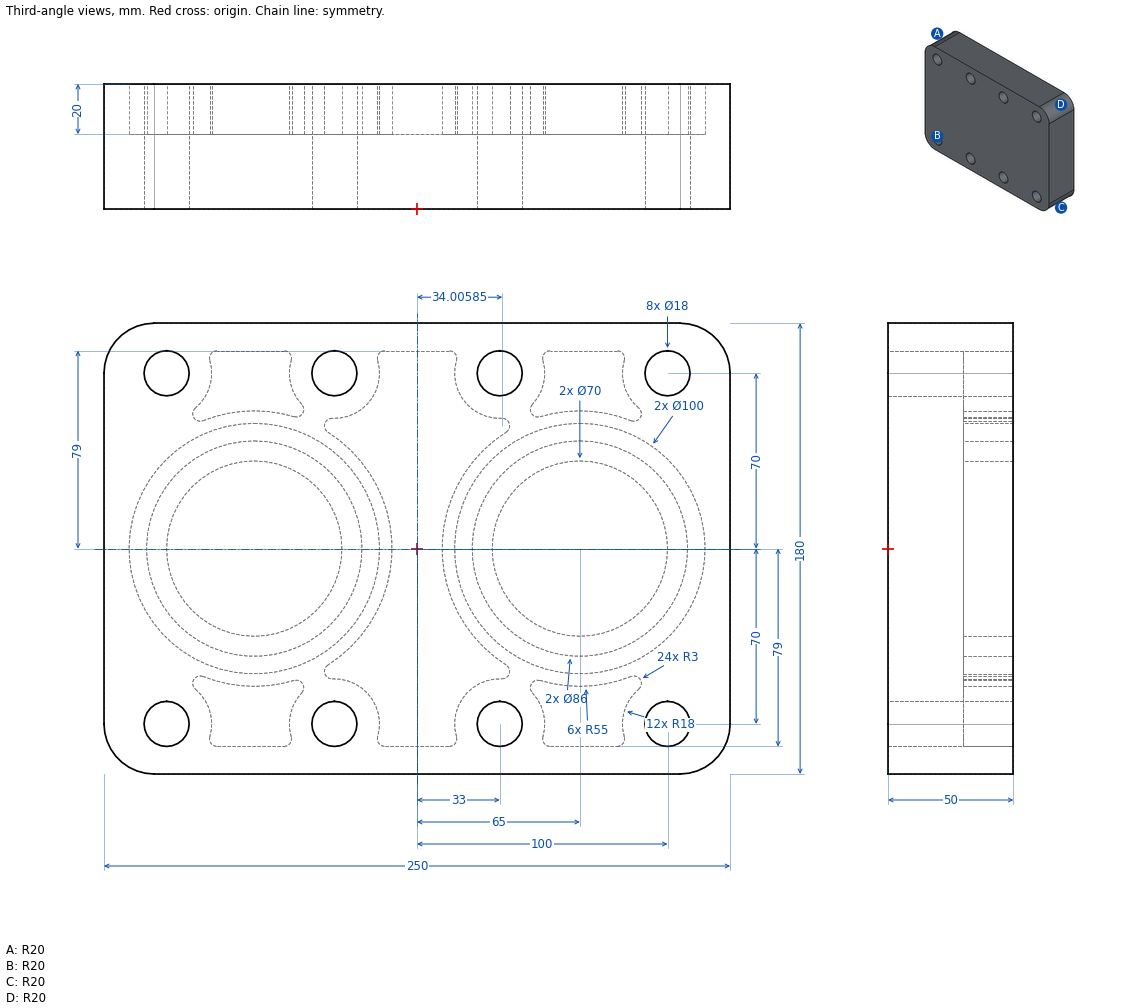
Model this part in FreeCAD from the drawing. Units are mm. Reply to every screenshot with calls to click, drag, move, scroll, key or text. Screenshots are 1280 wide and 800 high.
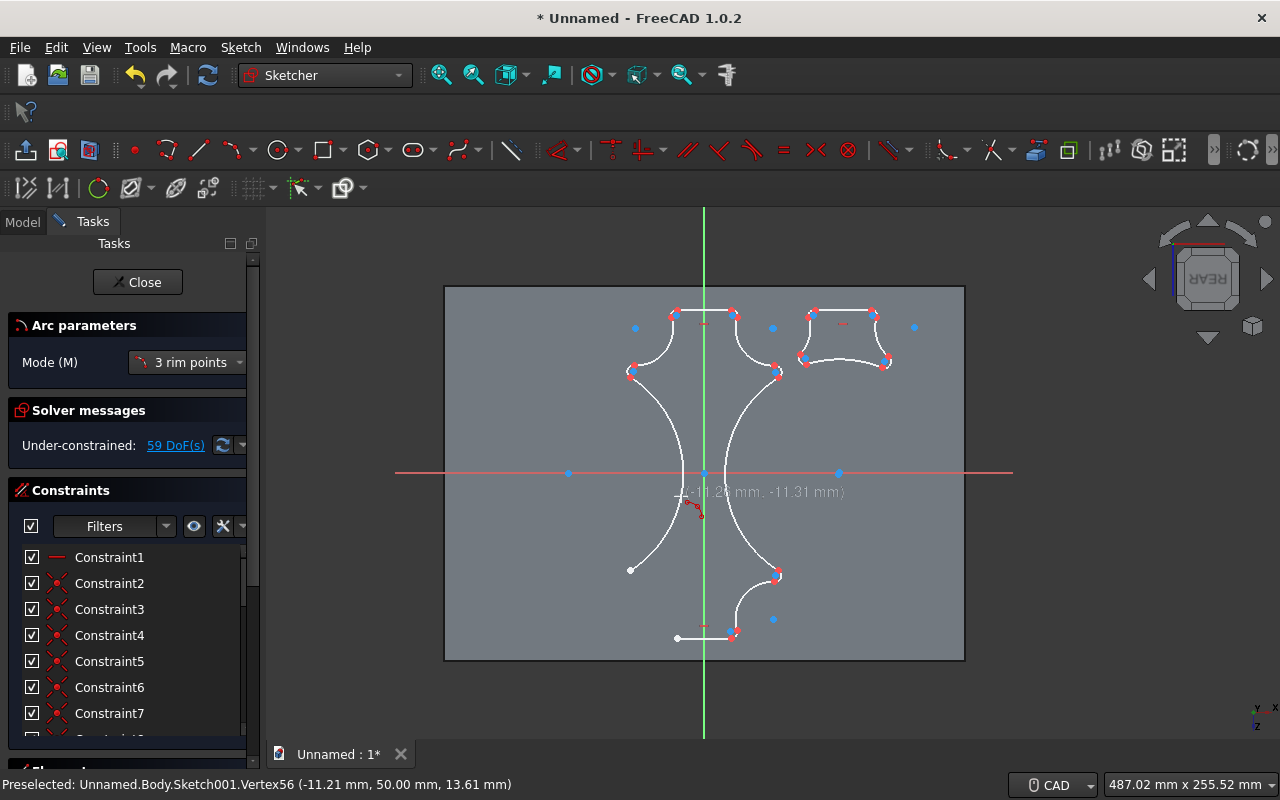
click(630, 571)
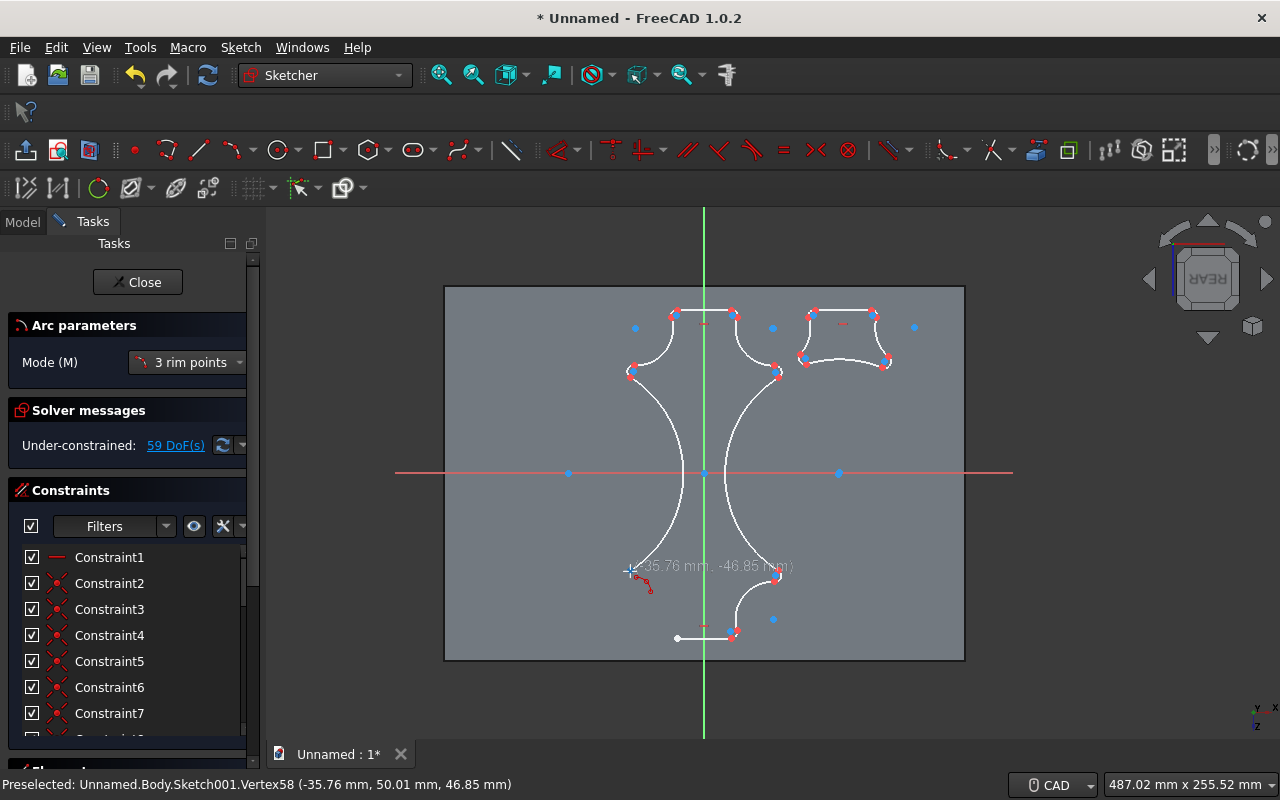
scroll(634, 582, up, 2)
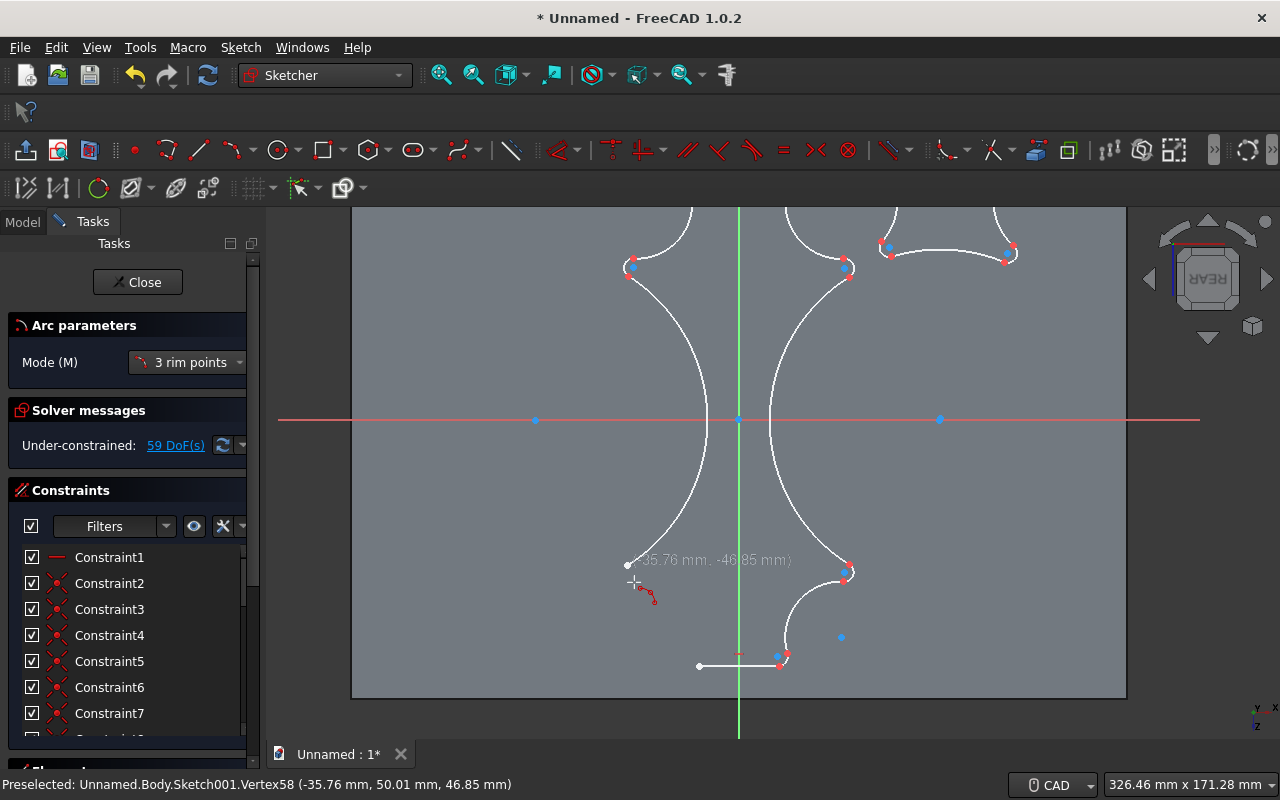
click(634, 581)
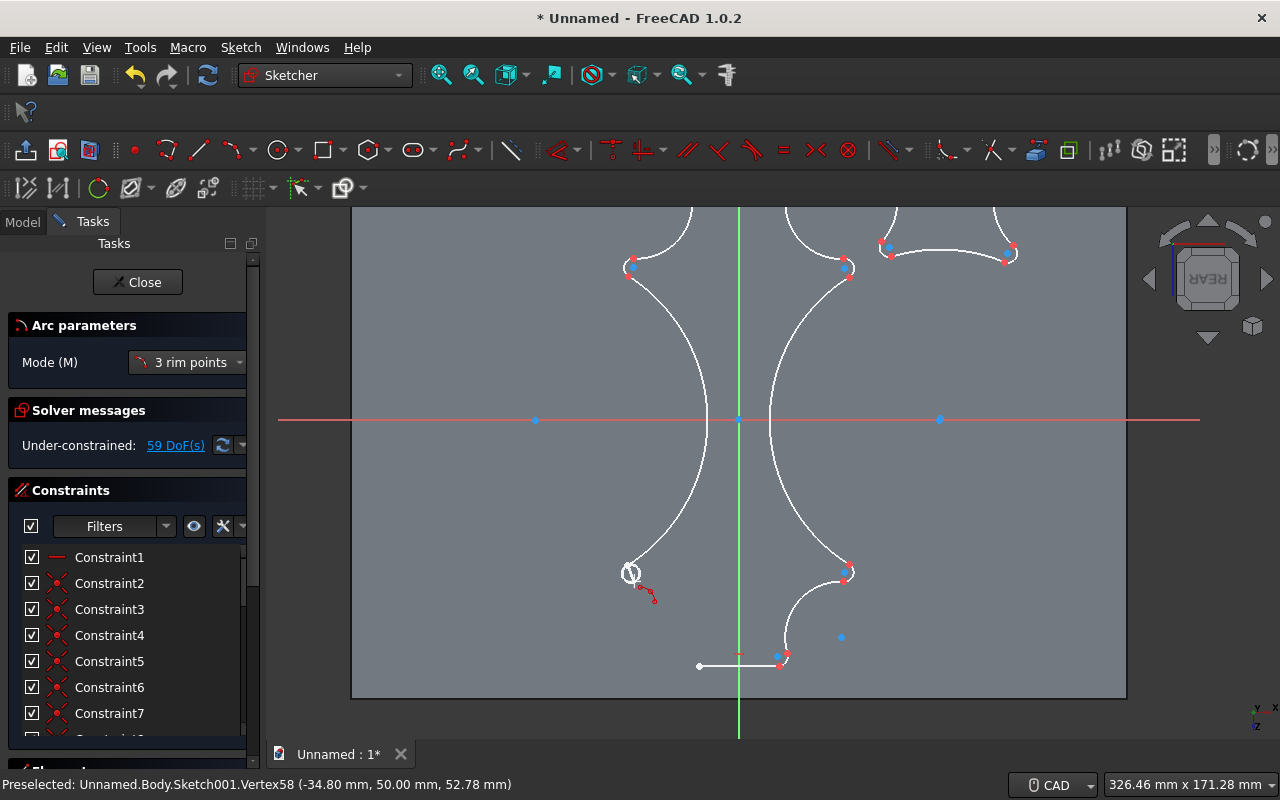
scroll(624, 575, up, 5)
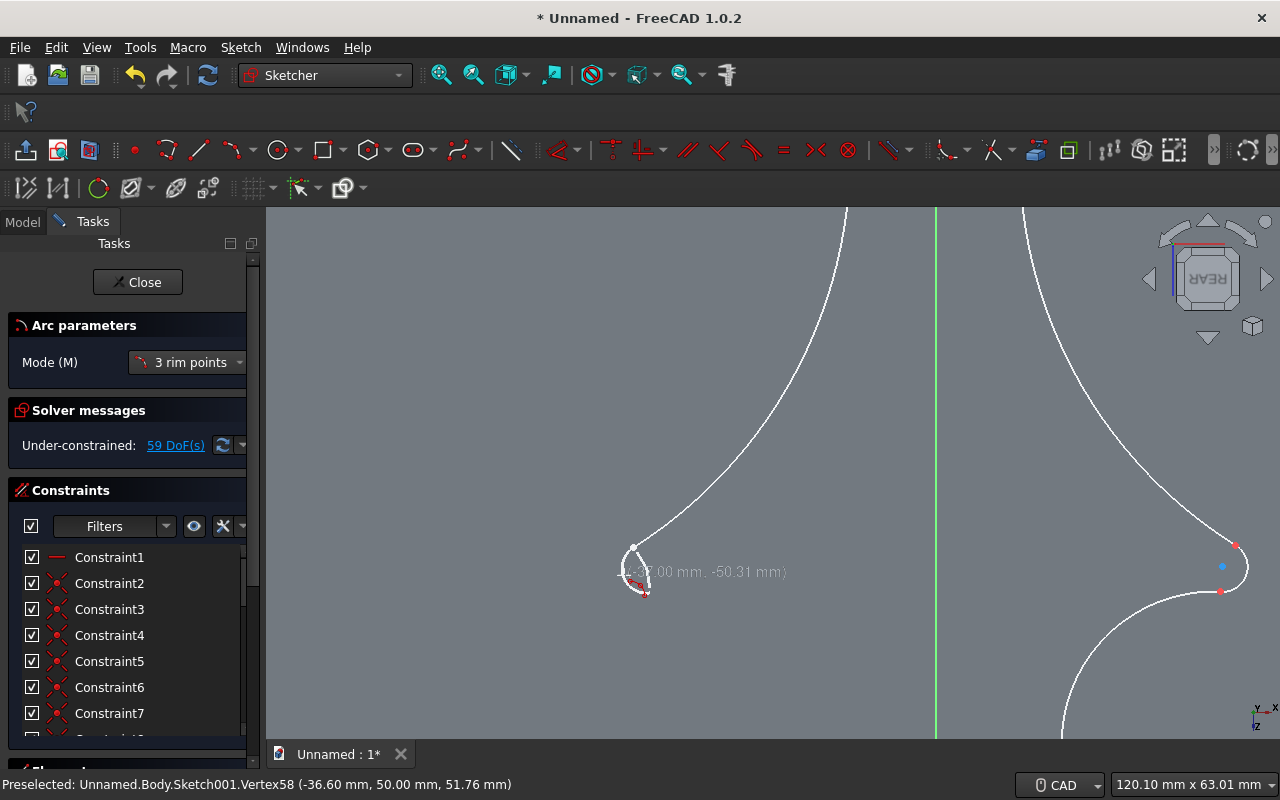
click(624, 573)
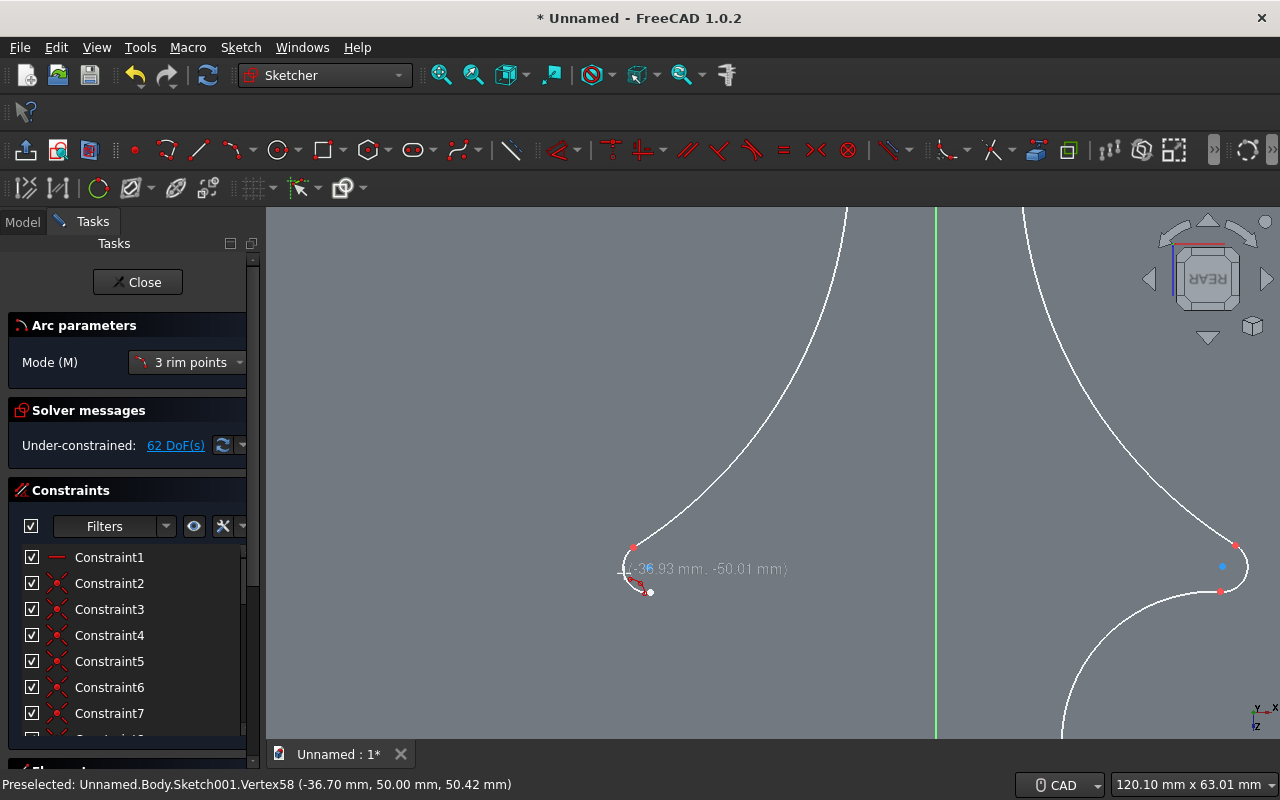
click(651, 593)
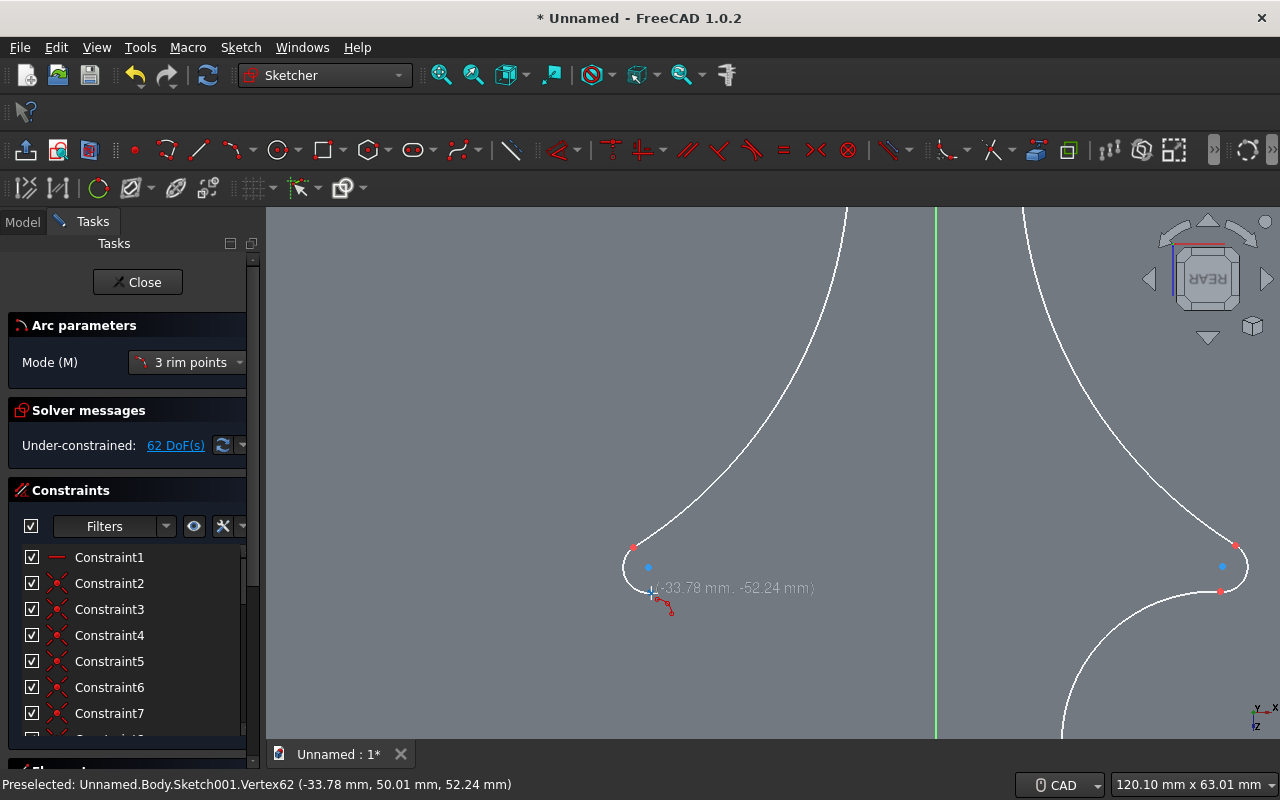
scroll(629, 578, down, 7)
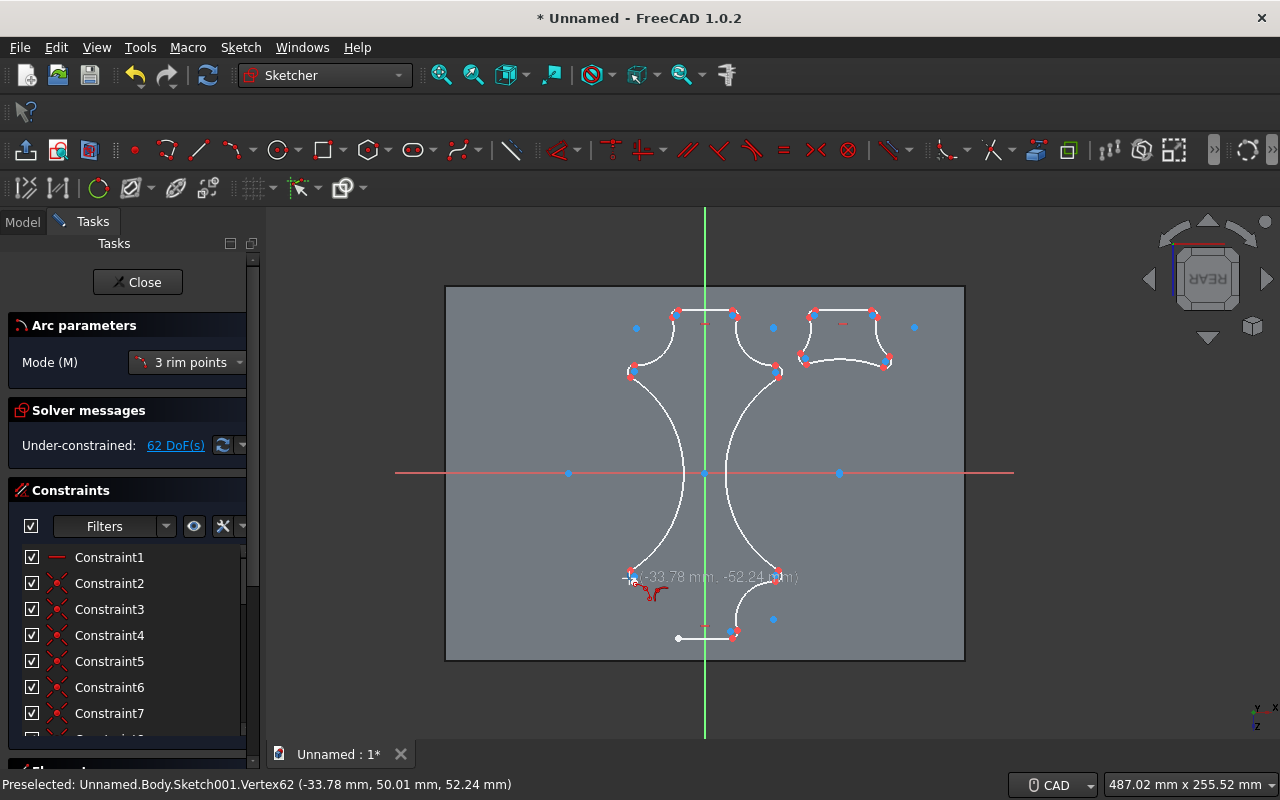
scroll(672, 630, up, 3)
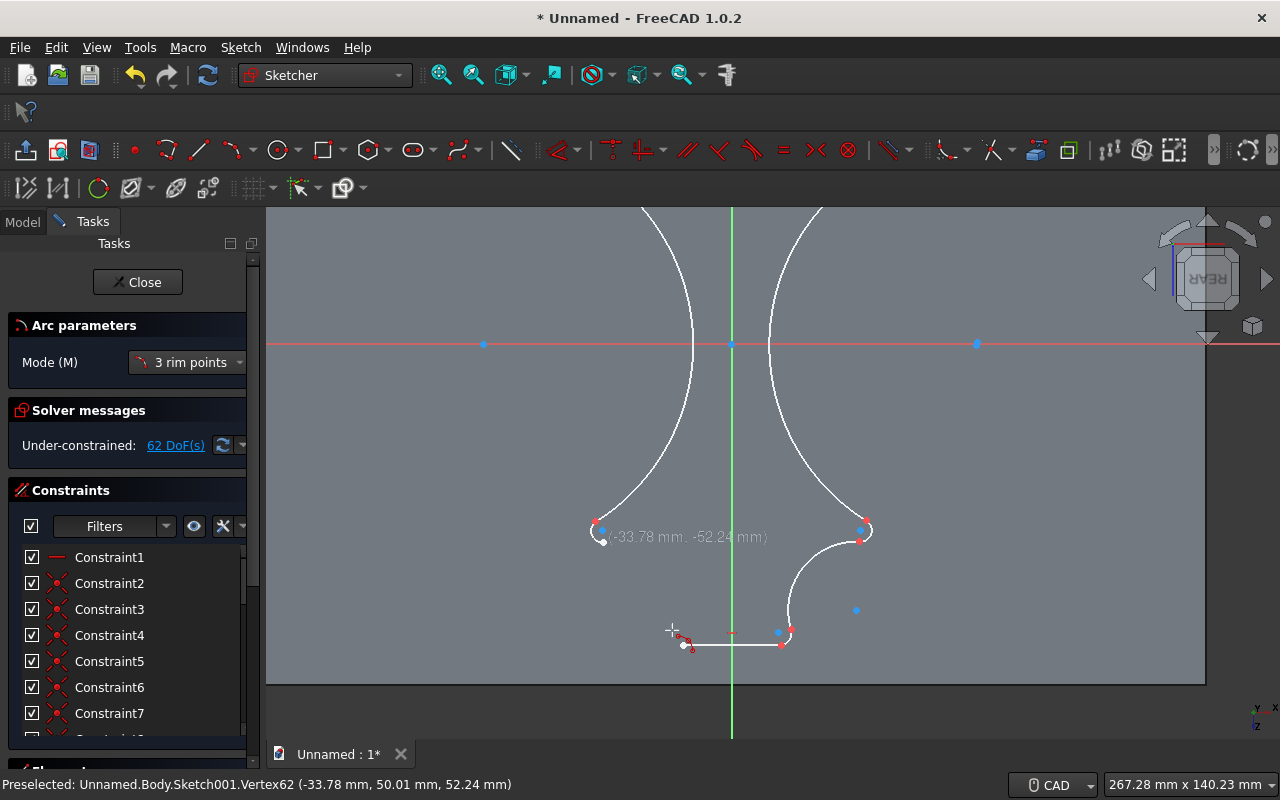
click(672, 629)
click(660, 567)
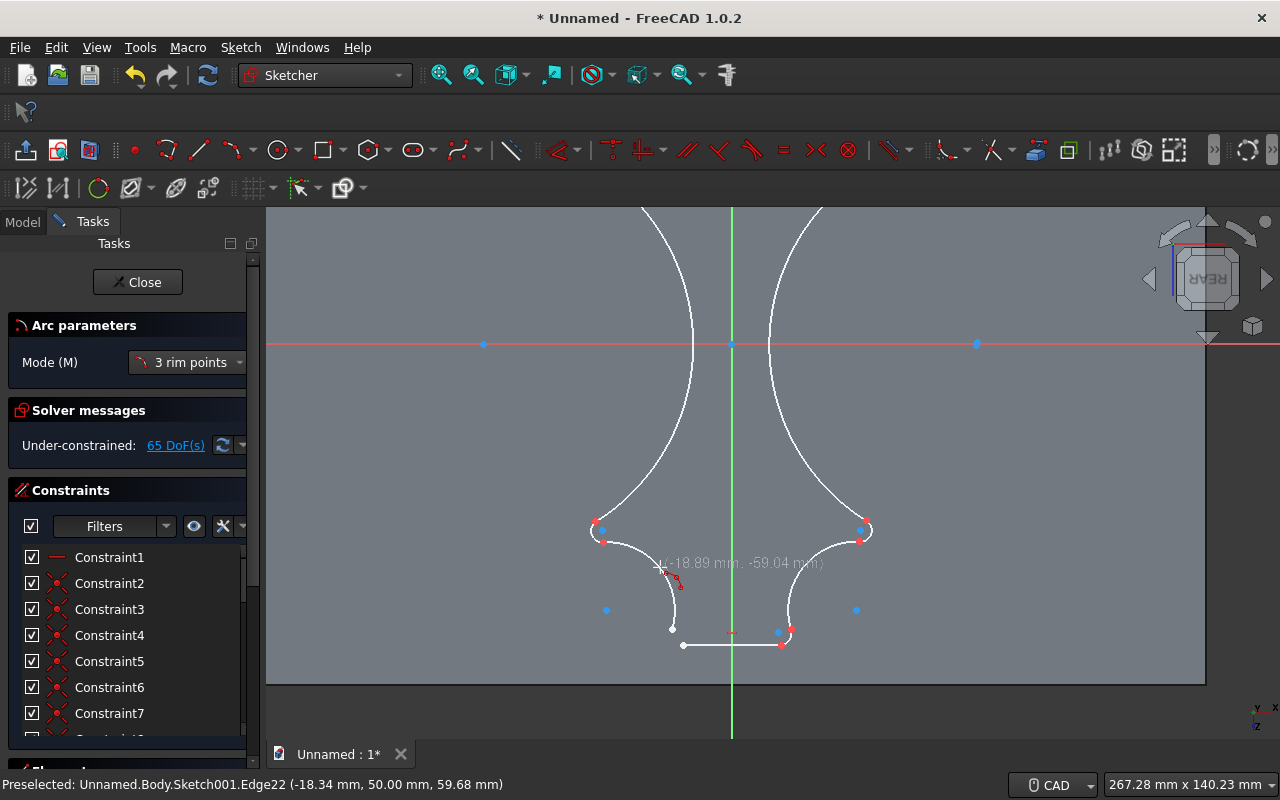
click(672, 630)
click(683, 645)